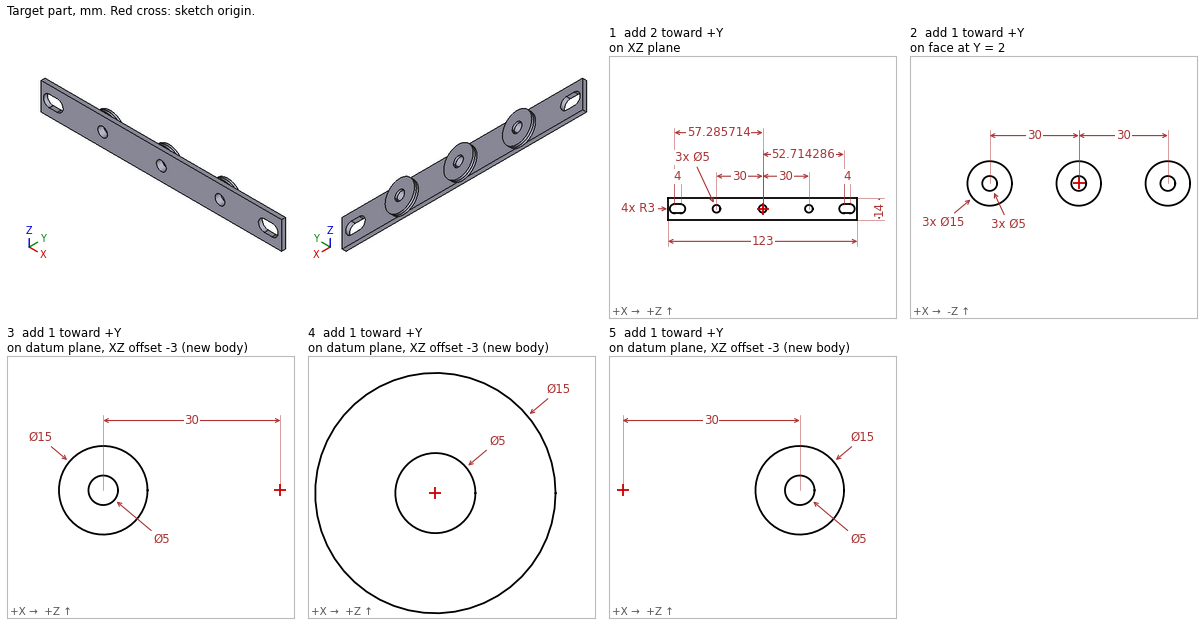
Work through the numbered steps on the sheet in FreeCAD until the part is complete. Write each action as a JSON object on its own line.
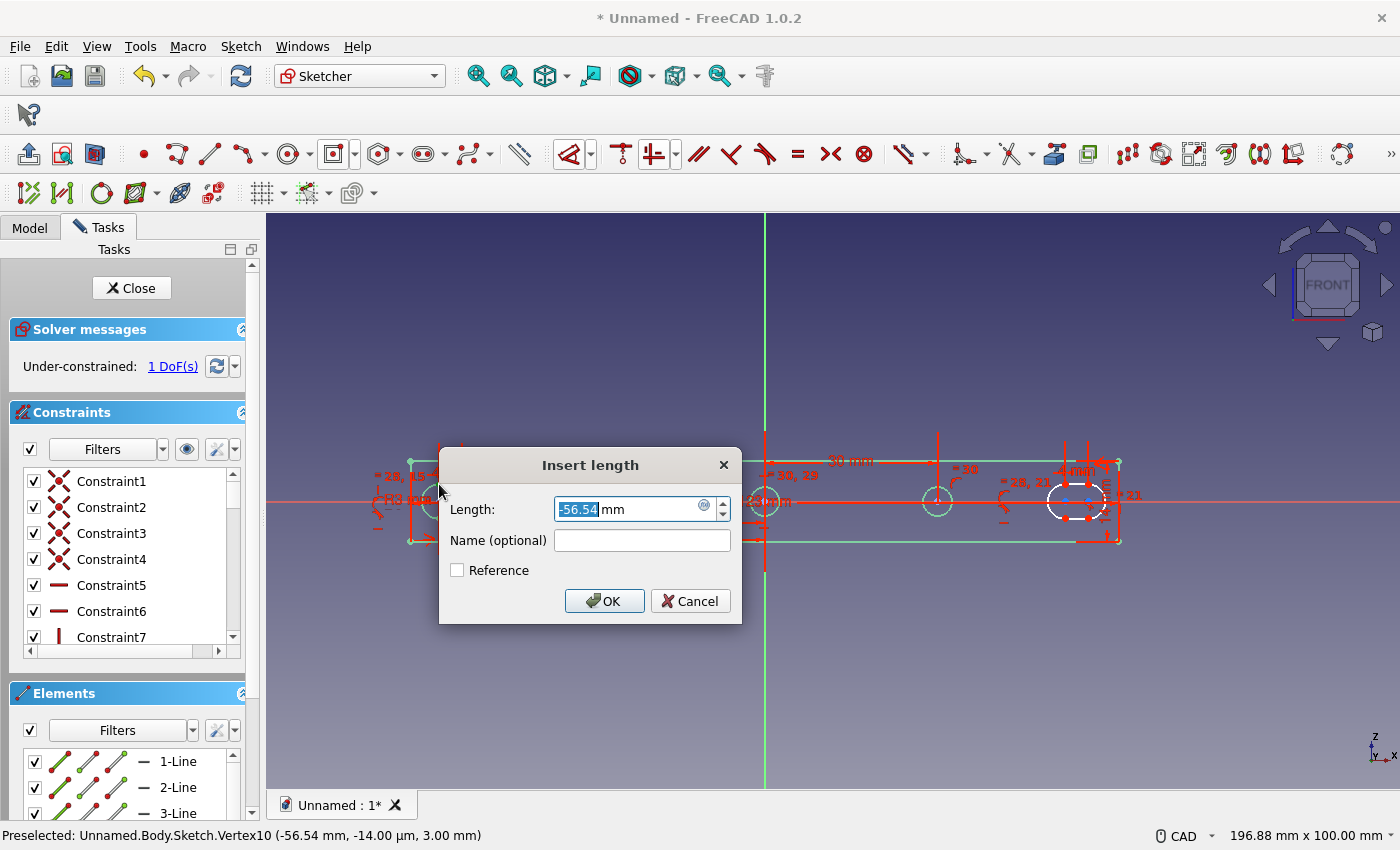
{"action": "type", "text": "-57.285714"}
{"action": "key", "text": "Return"}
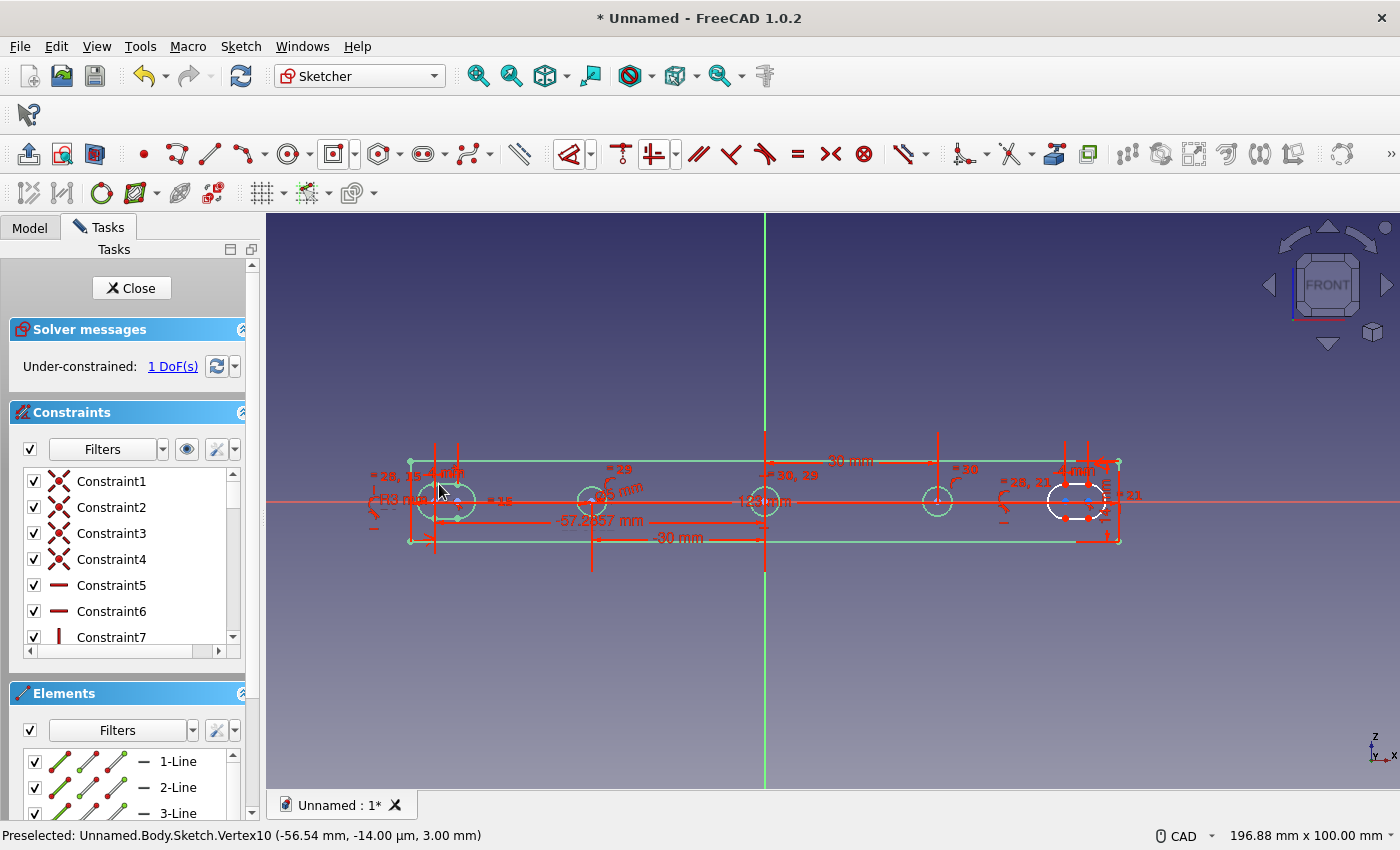
{"action": "left_click", "coordinate": [1065, 484]}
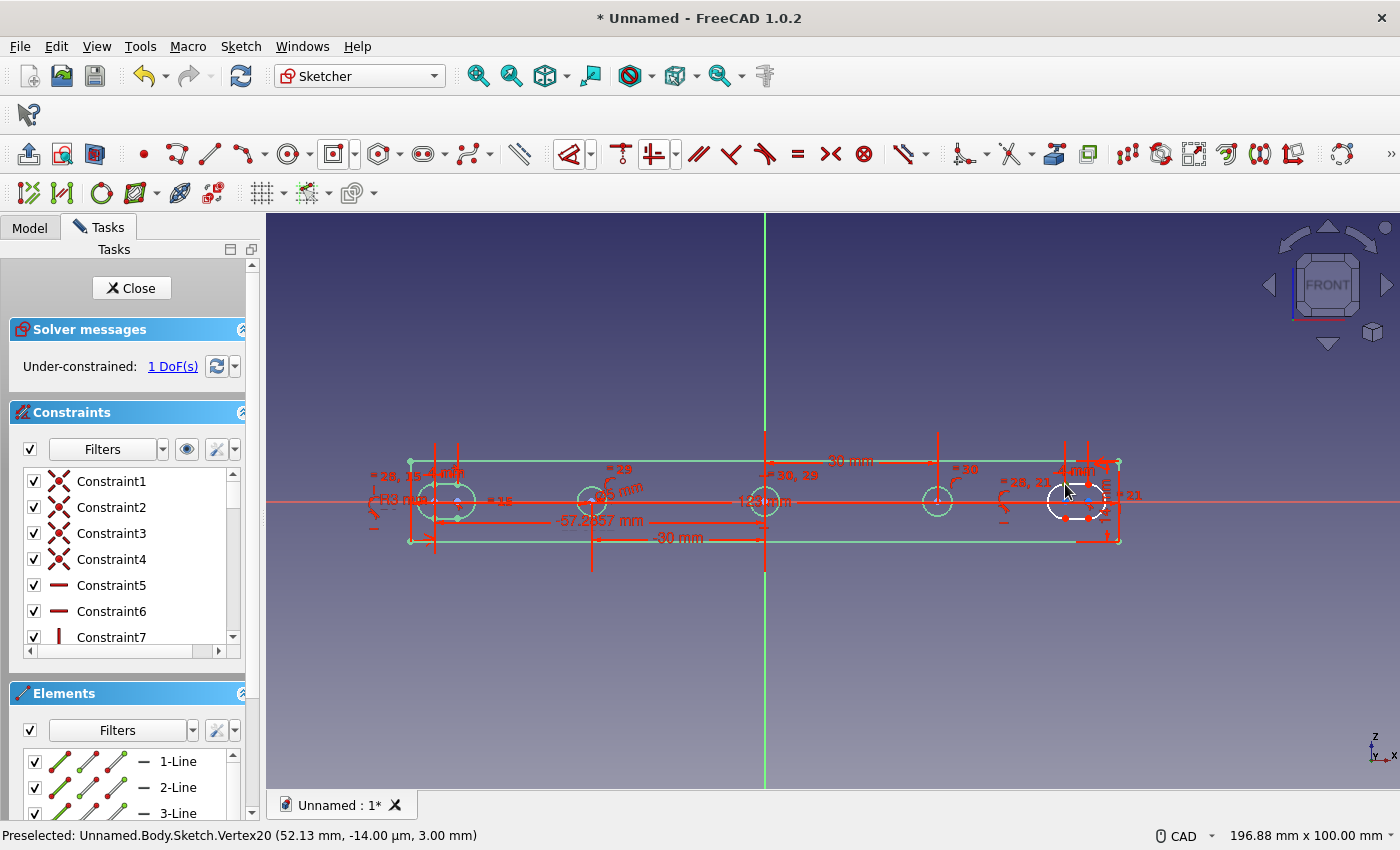
{"action": "key", "text": "l"}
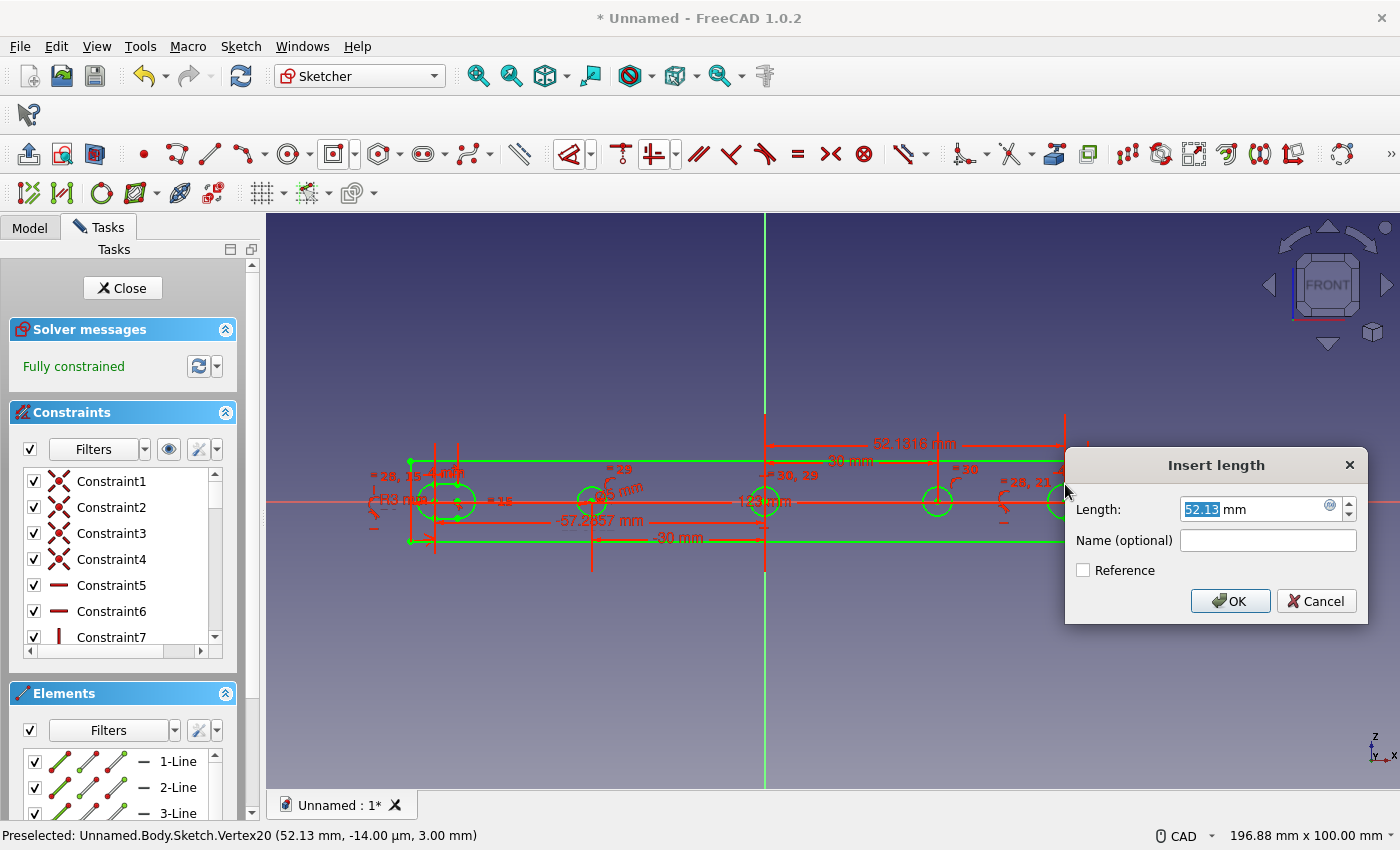
{"action": "type", "text": "52.714286"}
{"action": "key", "text": "Return"}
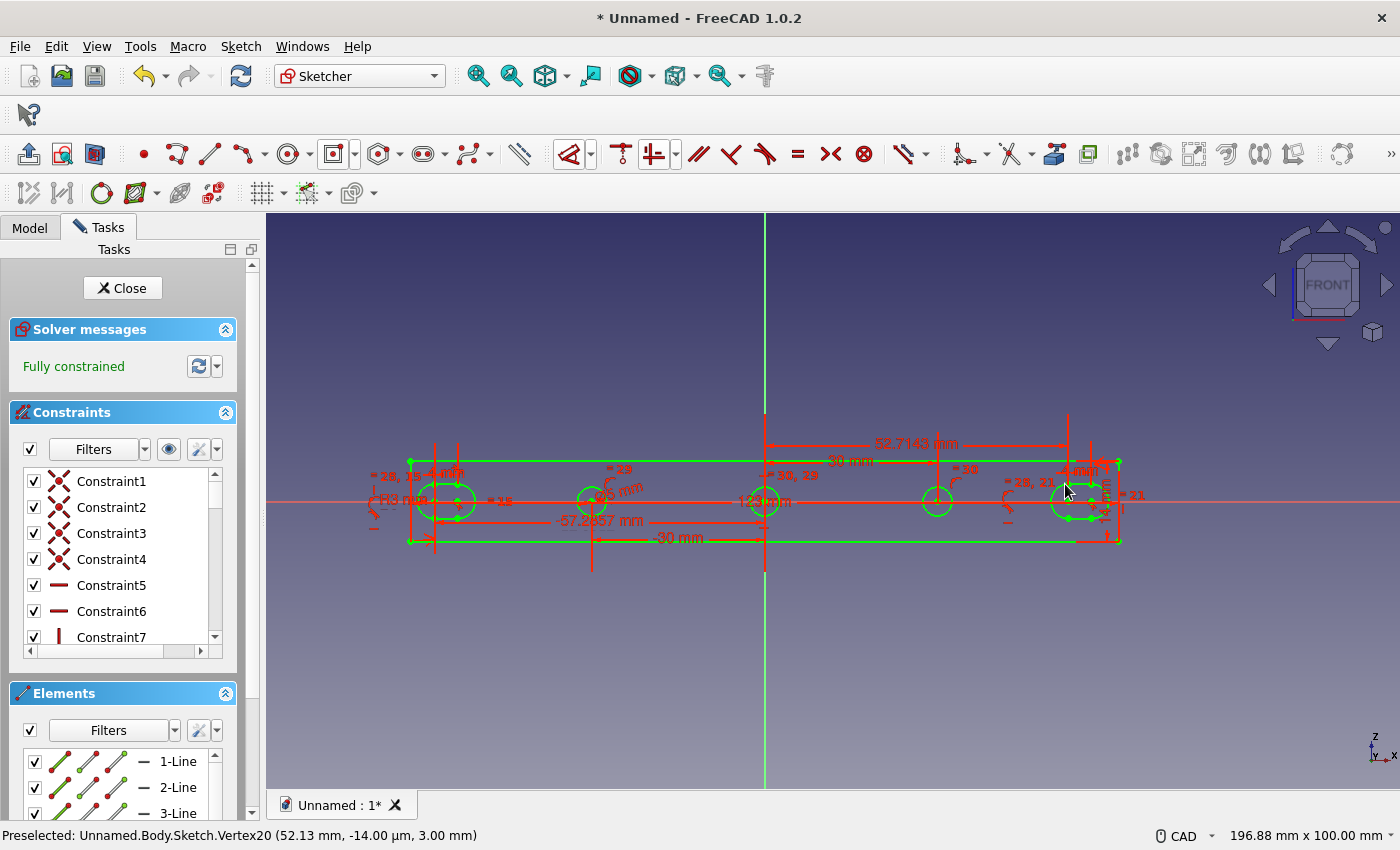
{"action": "left_click", "coordinate": [123, 288]}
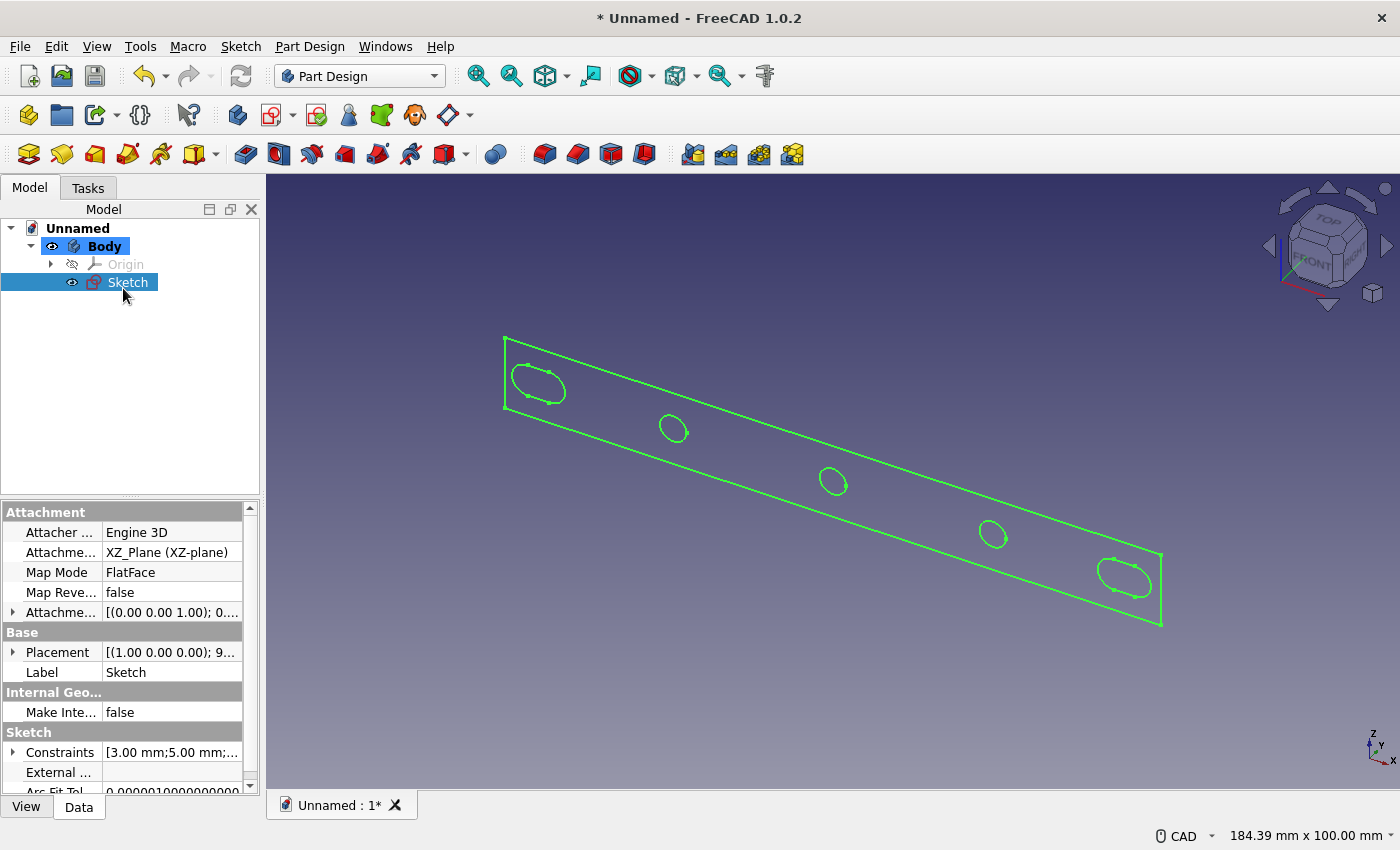
{"action": "left_click", "coordinate": [29, 154]}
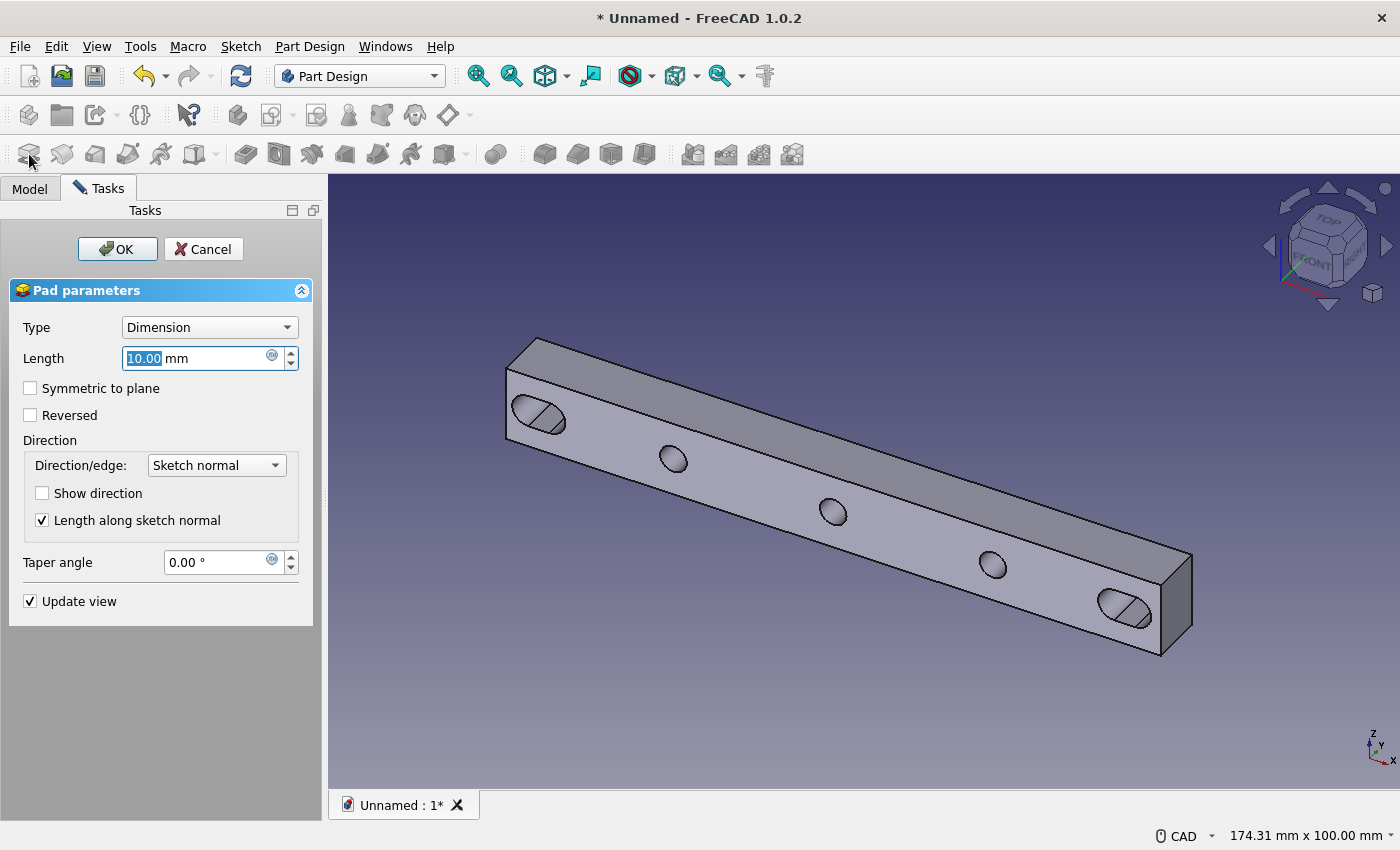
{"action": "type", "text": "2"}
{"action": "key", "text": "Tab"}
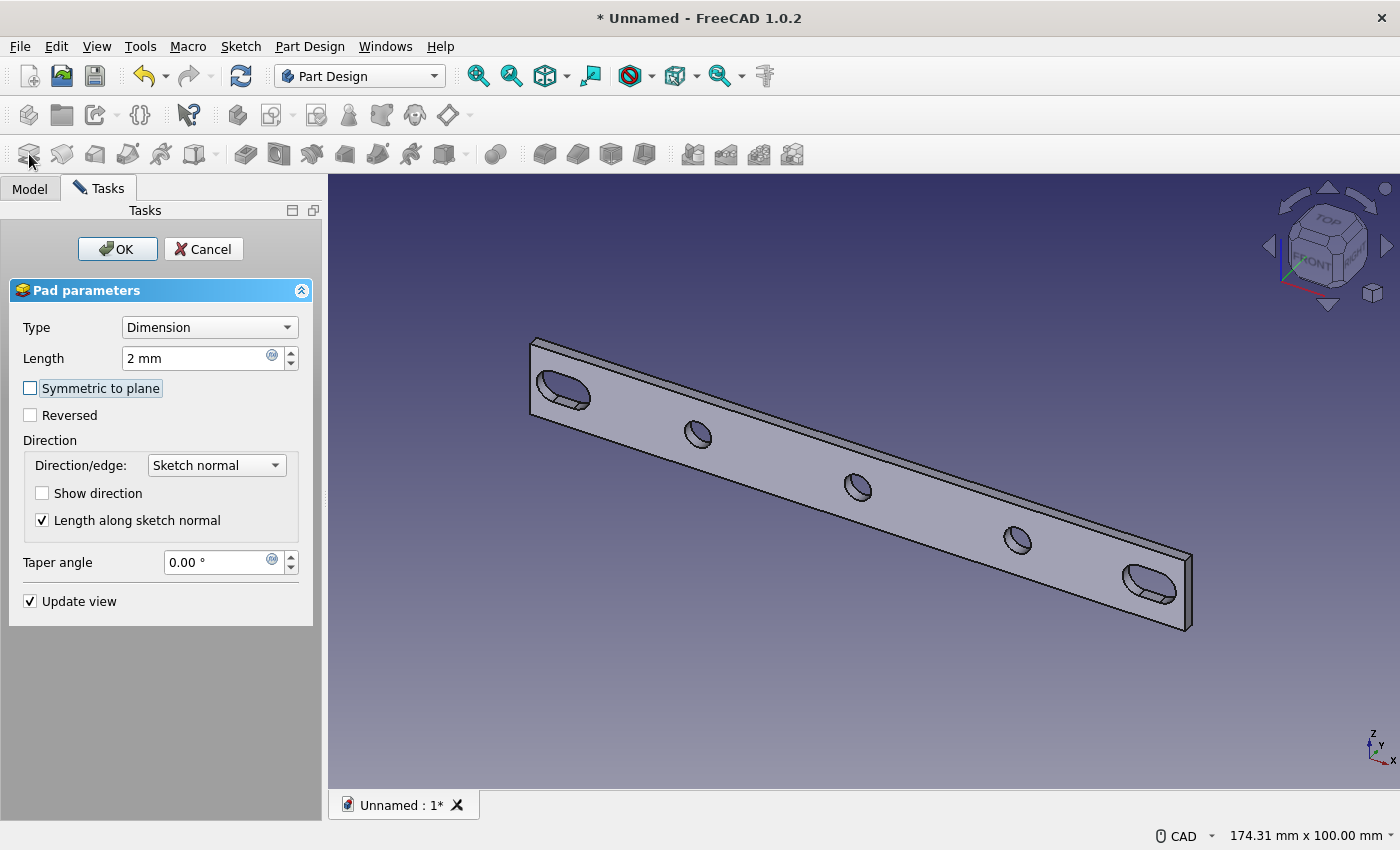
{"action": "left_click", "coordinate": [31, 415]}